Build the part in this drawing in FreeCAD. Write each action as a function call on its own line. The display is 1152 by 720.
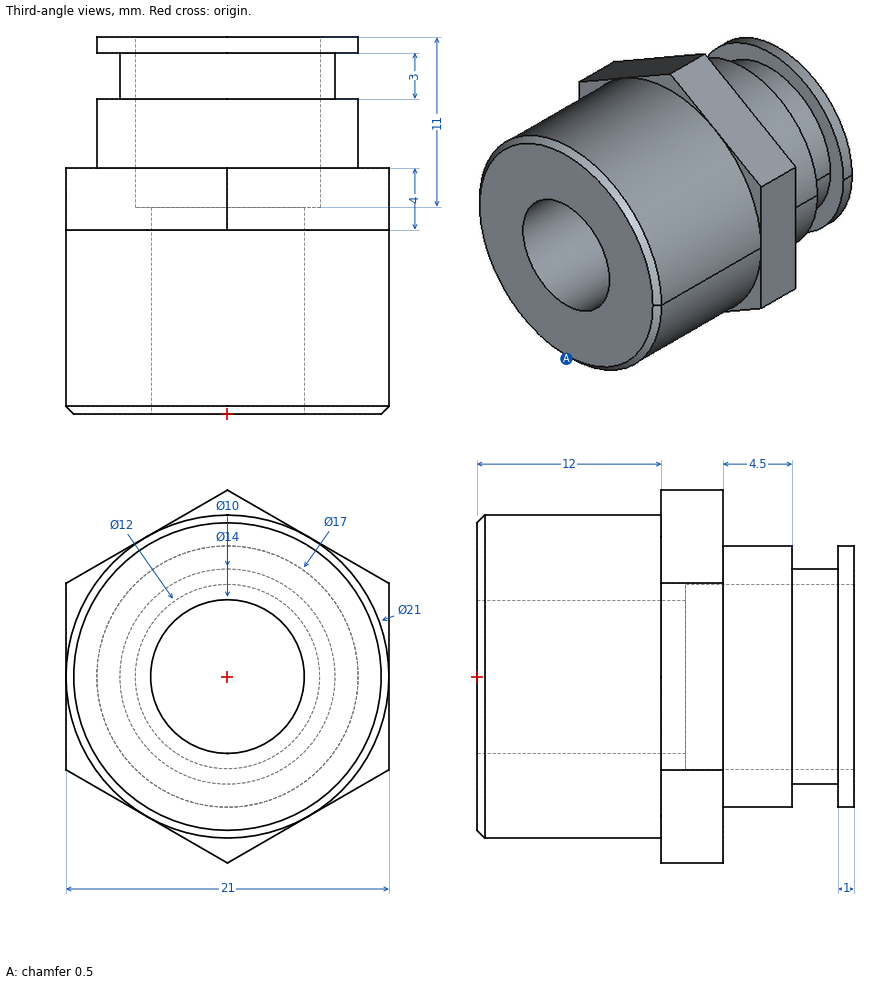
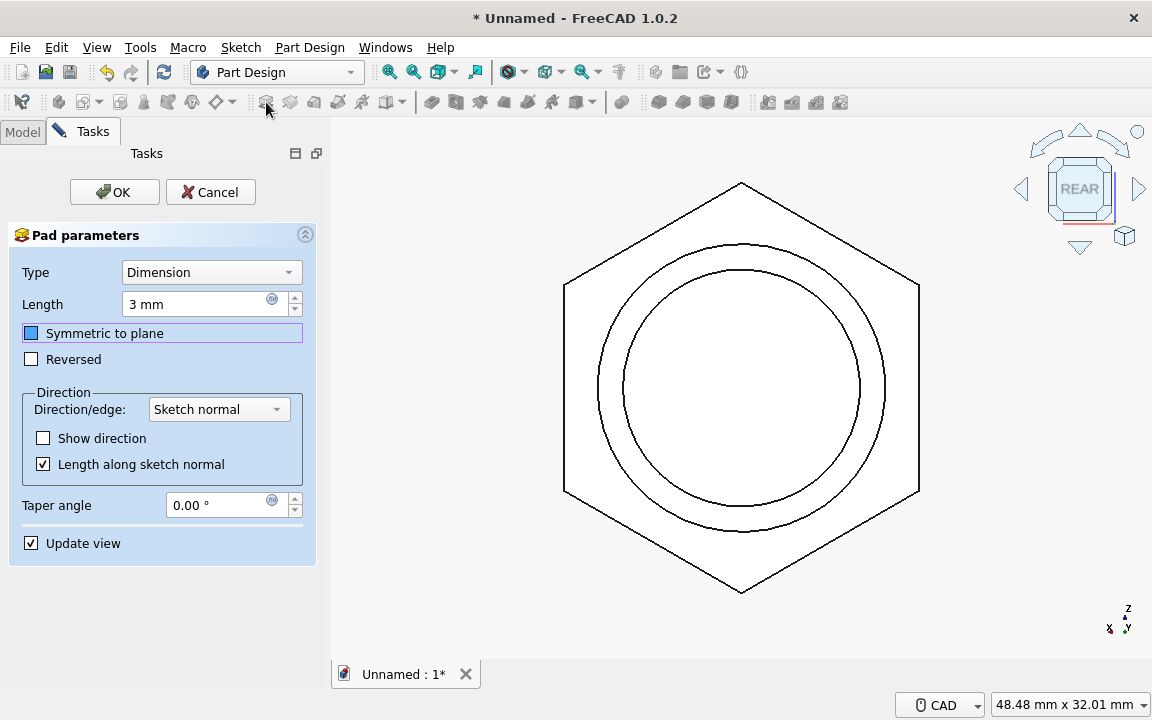
click(115, 192)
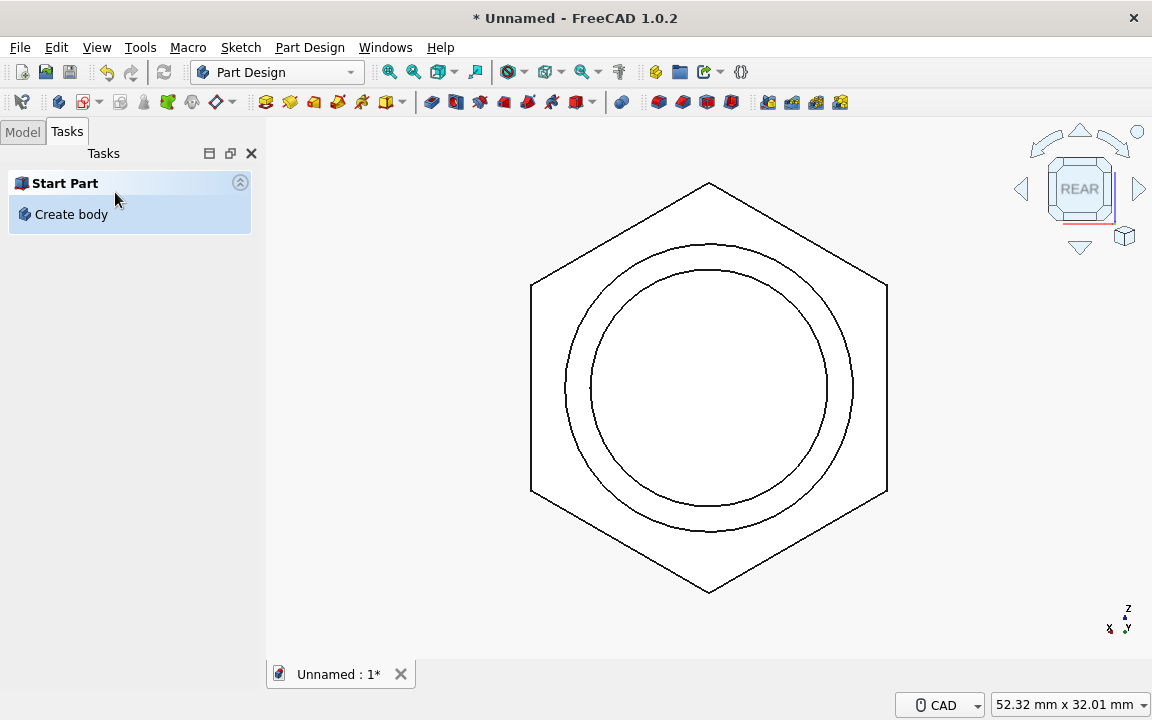
click(709, 387)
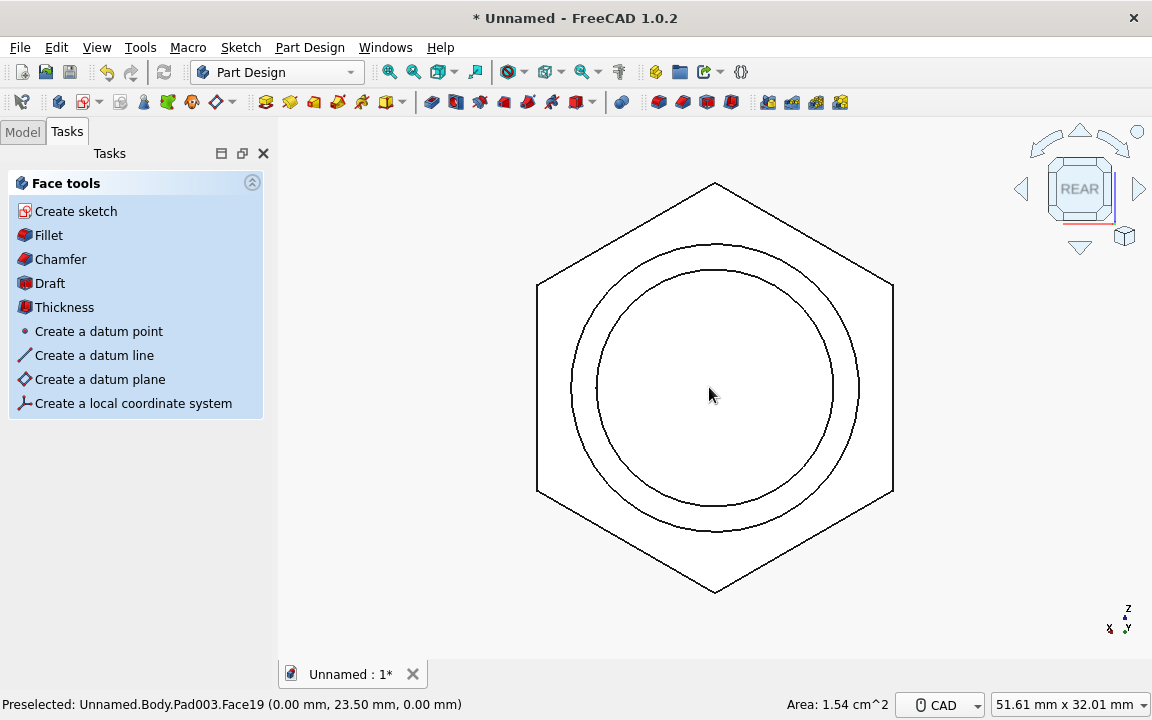
click(84, 102)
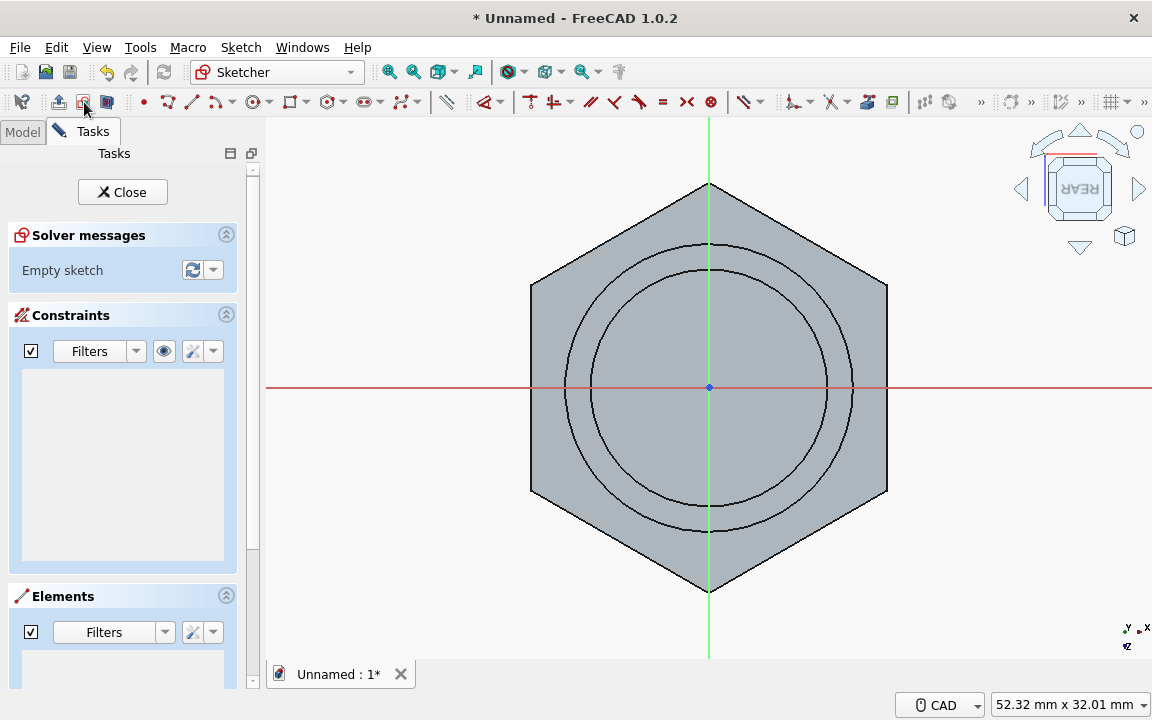
click(254, 102)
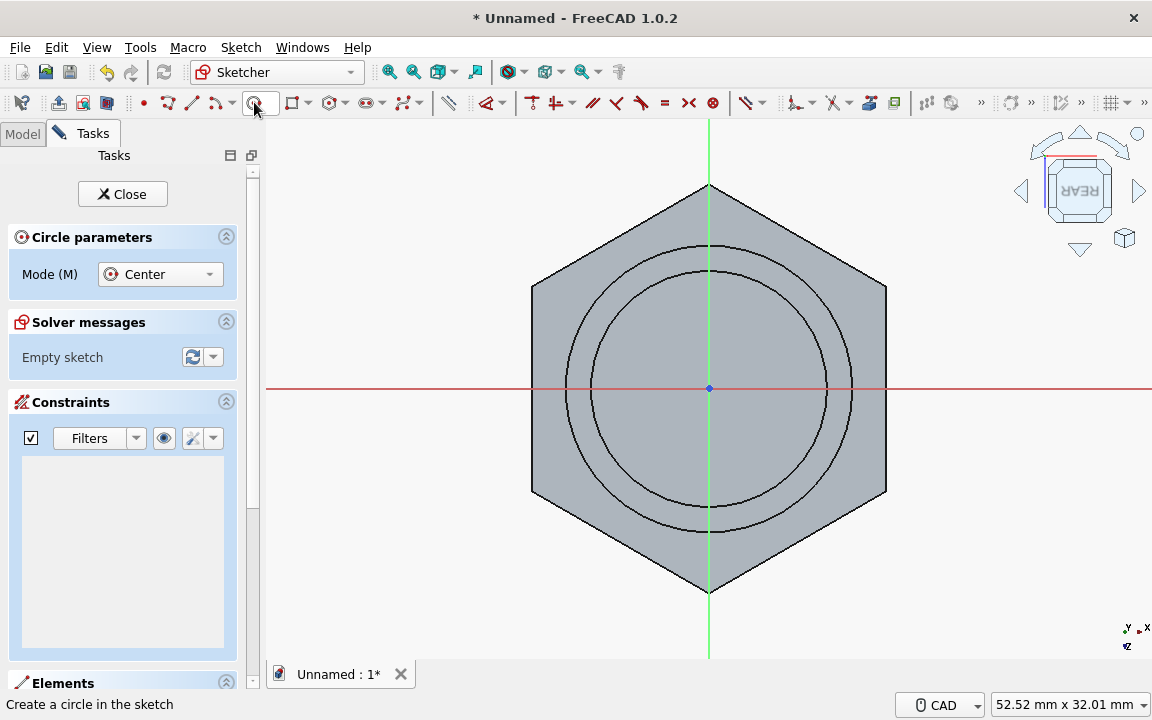
click(709, 389)
move(810, 288)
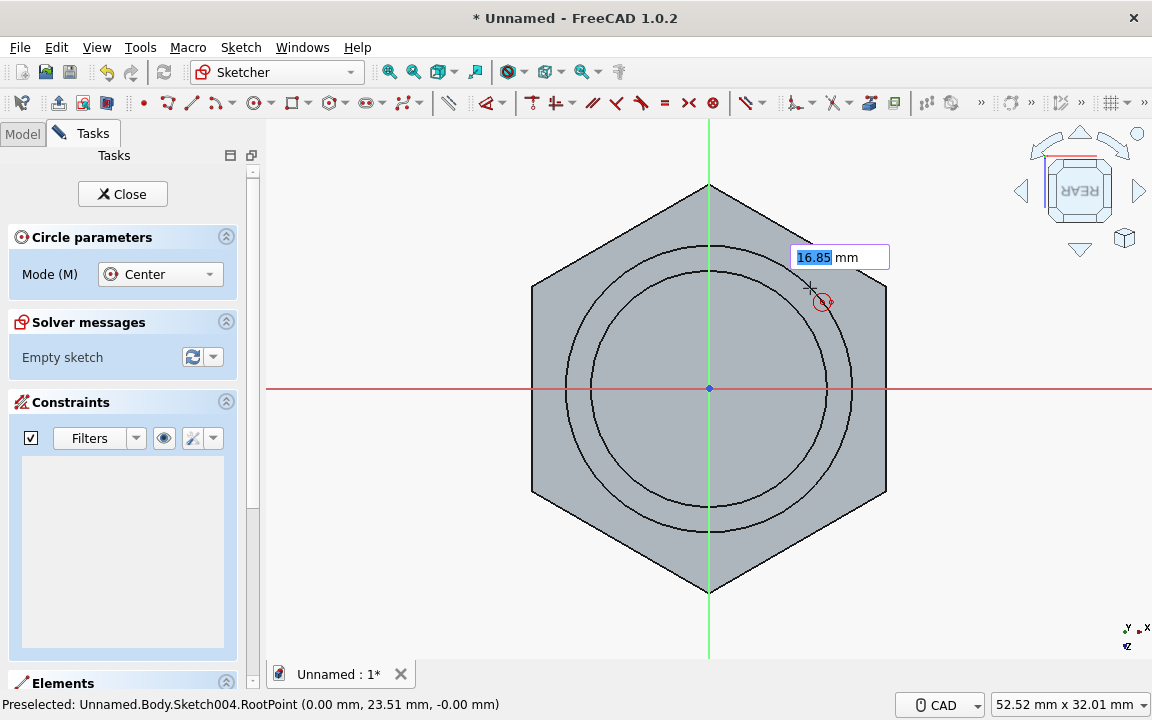
text(17)
key(Return)
key(Escape)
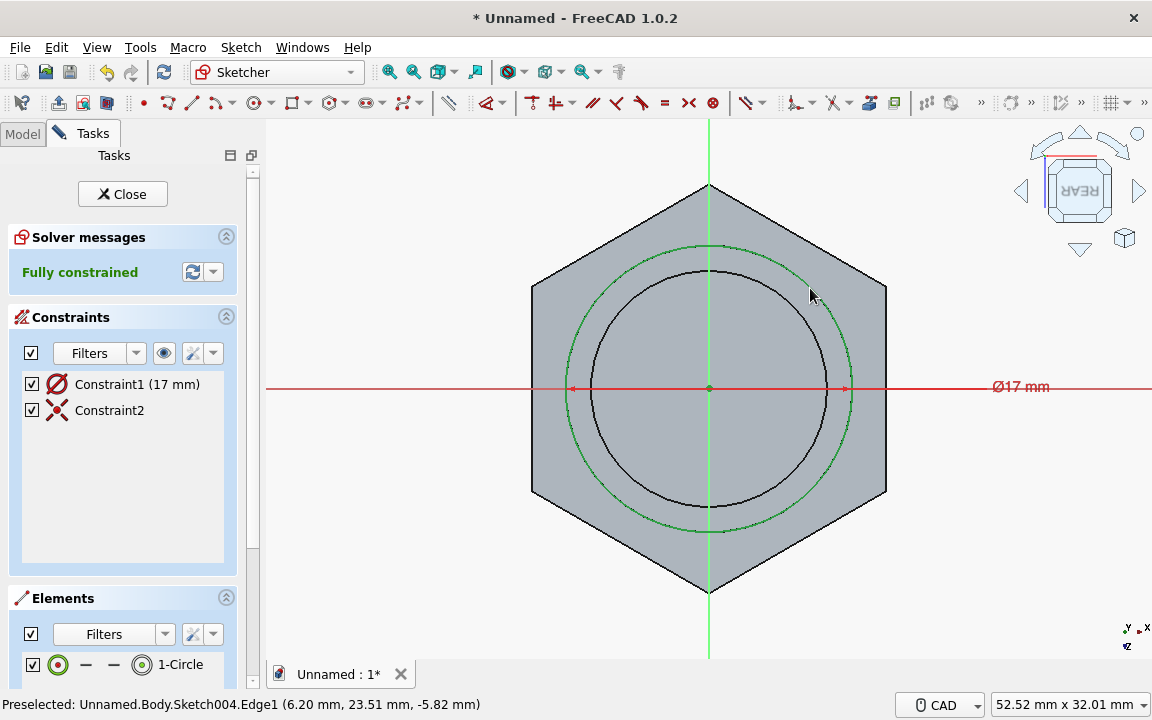
click(123, 194)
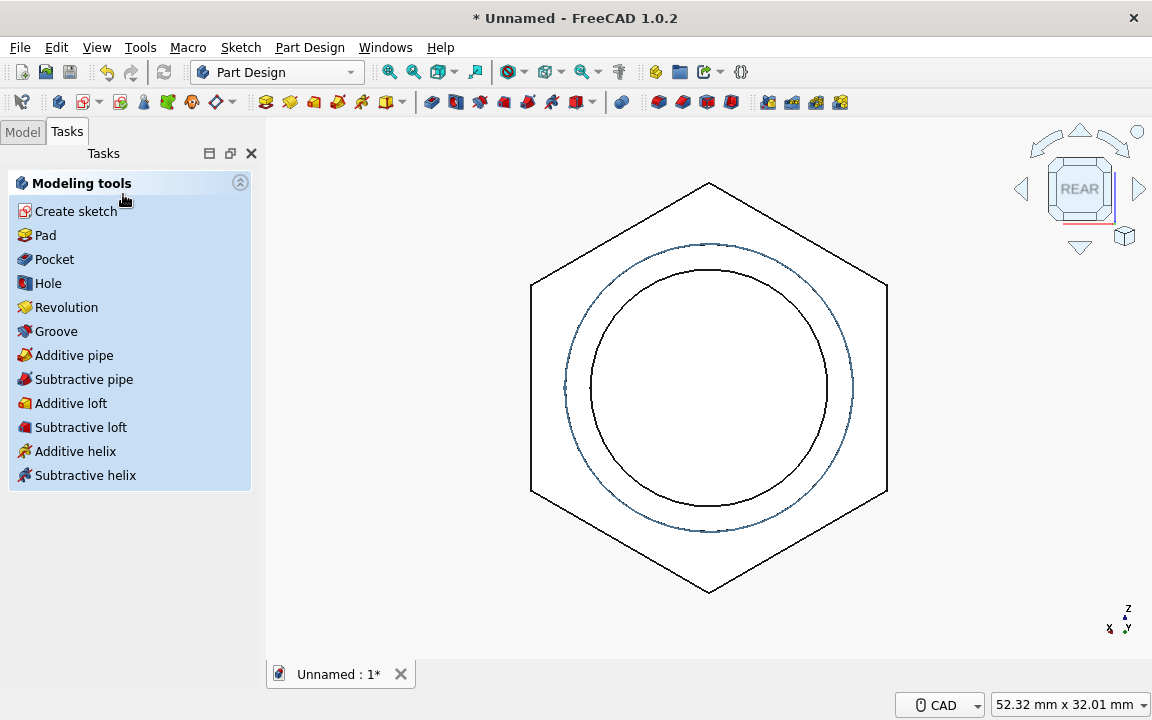
click(266, 102)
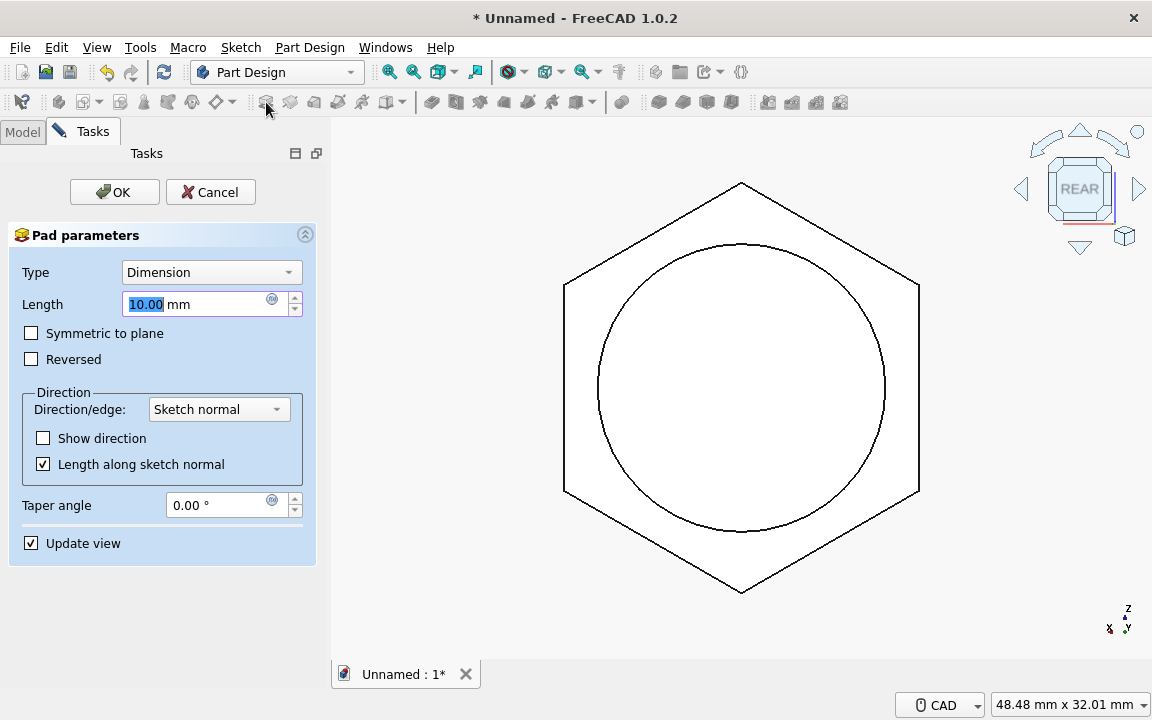
text(1)
key(Tab)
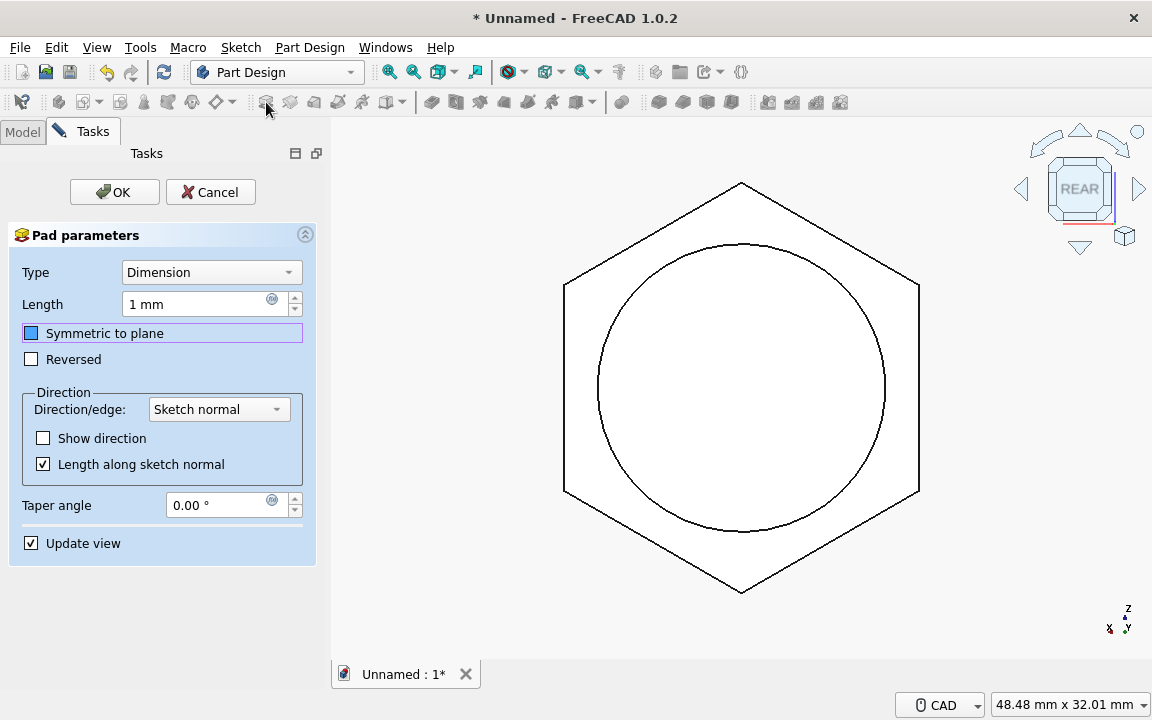
click(115, 192)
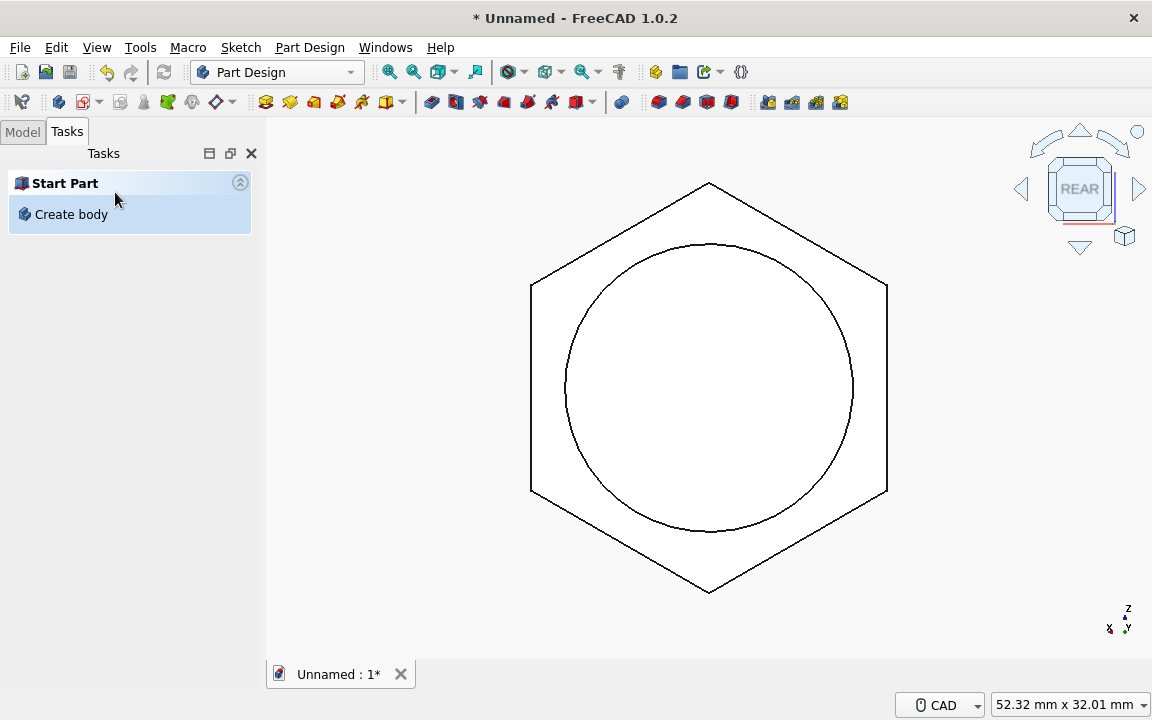
key(0)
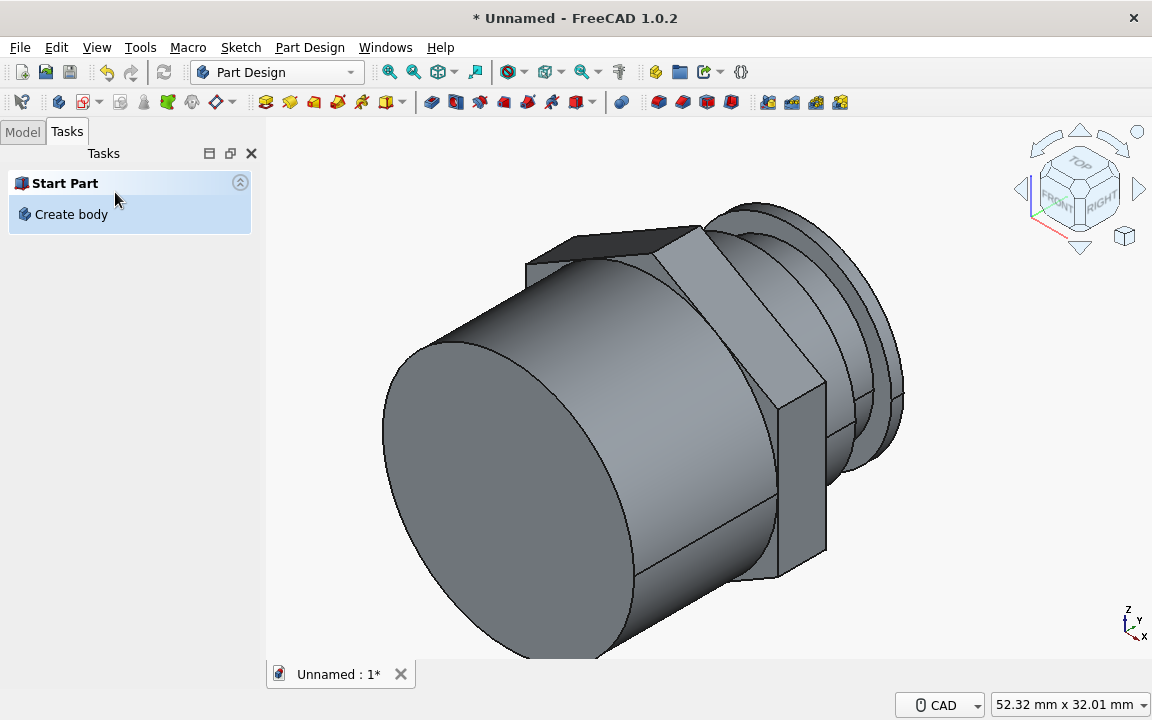
key(v)
key(f)